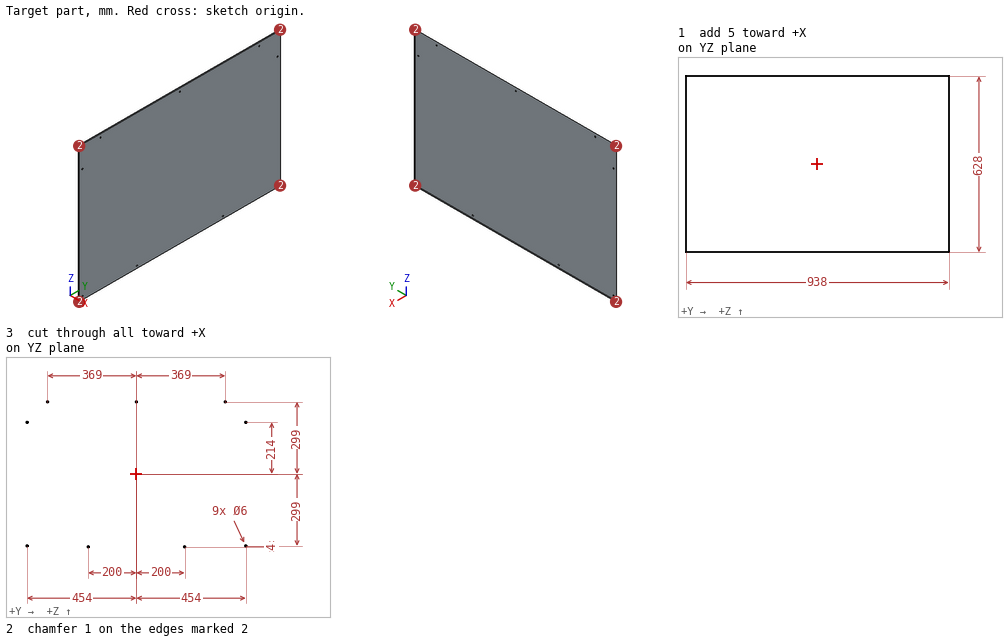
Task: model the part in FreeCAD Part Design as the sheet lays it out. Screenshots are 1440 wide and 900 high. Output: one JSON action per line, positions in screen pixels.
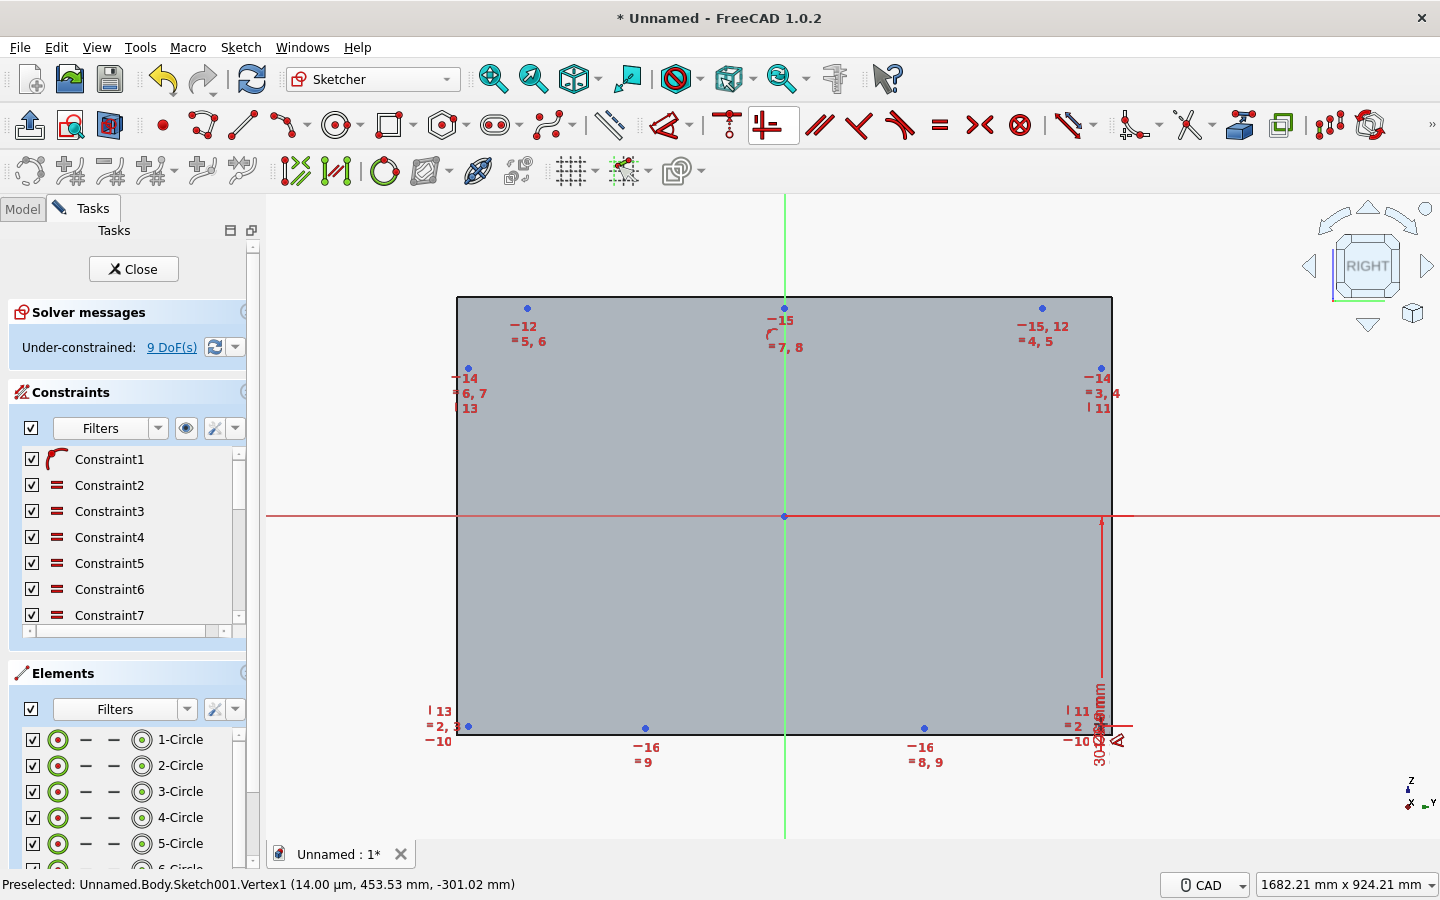
{"action": "scroll", "coordinate": [924, 728], "scroll_direction": "up", "scroll_amount": 14}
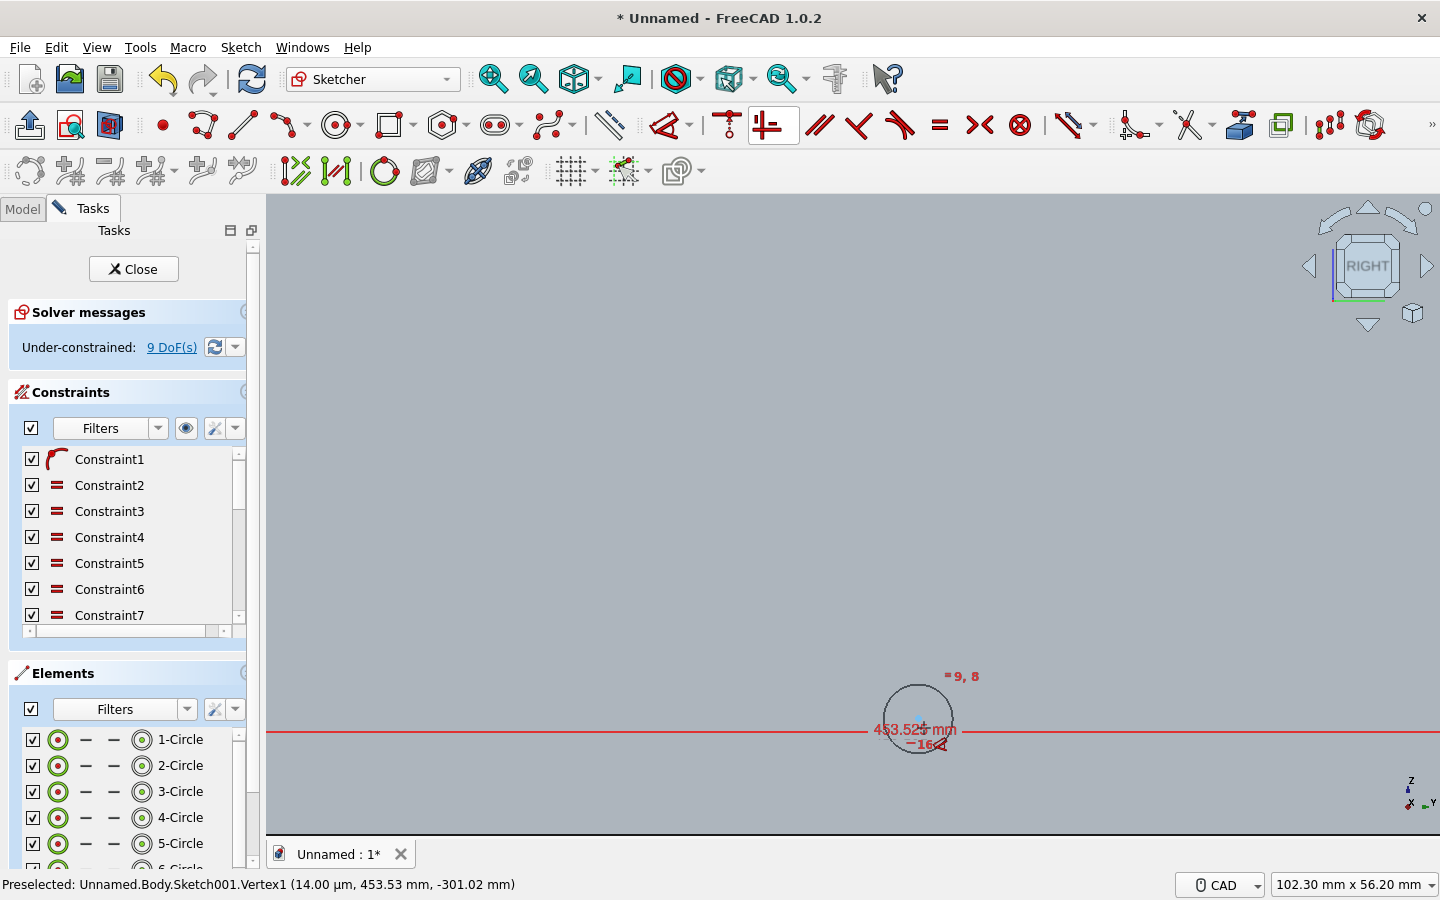
{"action": "left_click", "coordinate": [918, 719]}
{"action": "left_click", "coordinate": [860, 702]}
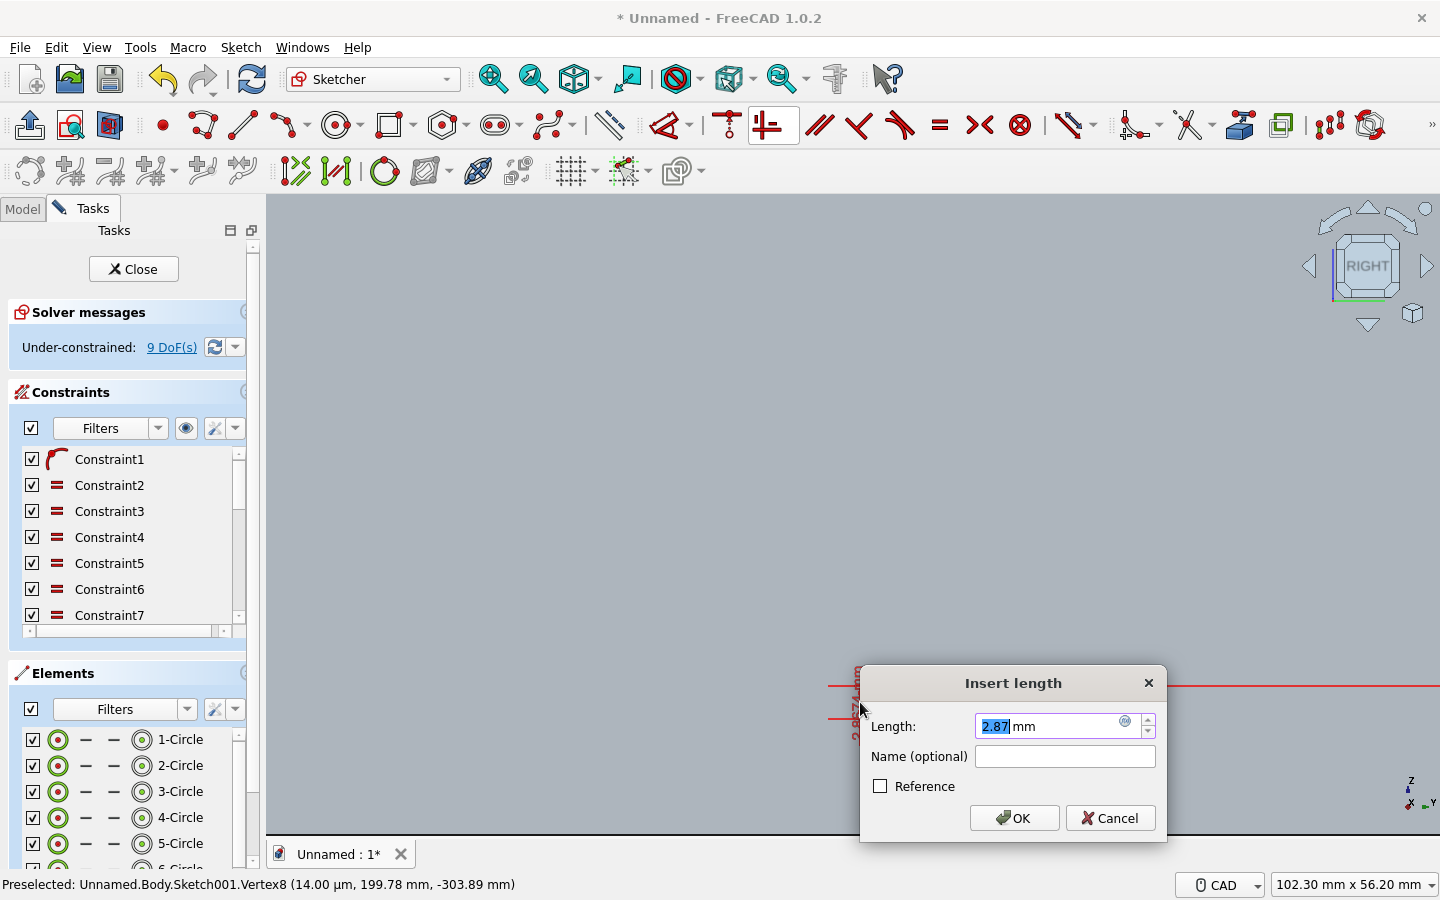
{"action": "type", "text": "4"}
{"action": "key", "text": "Return"}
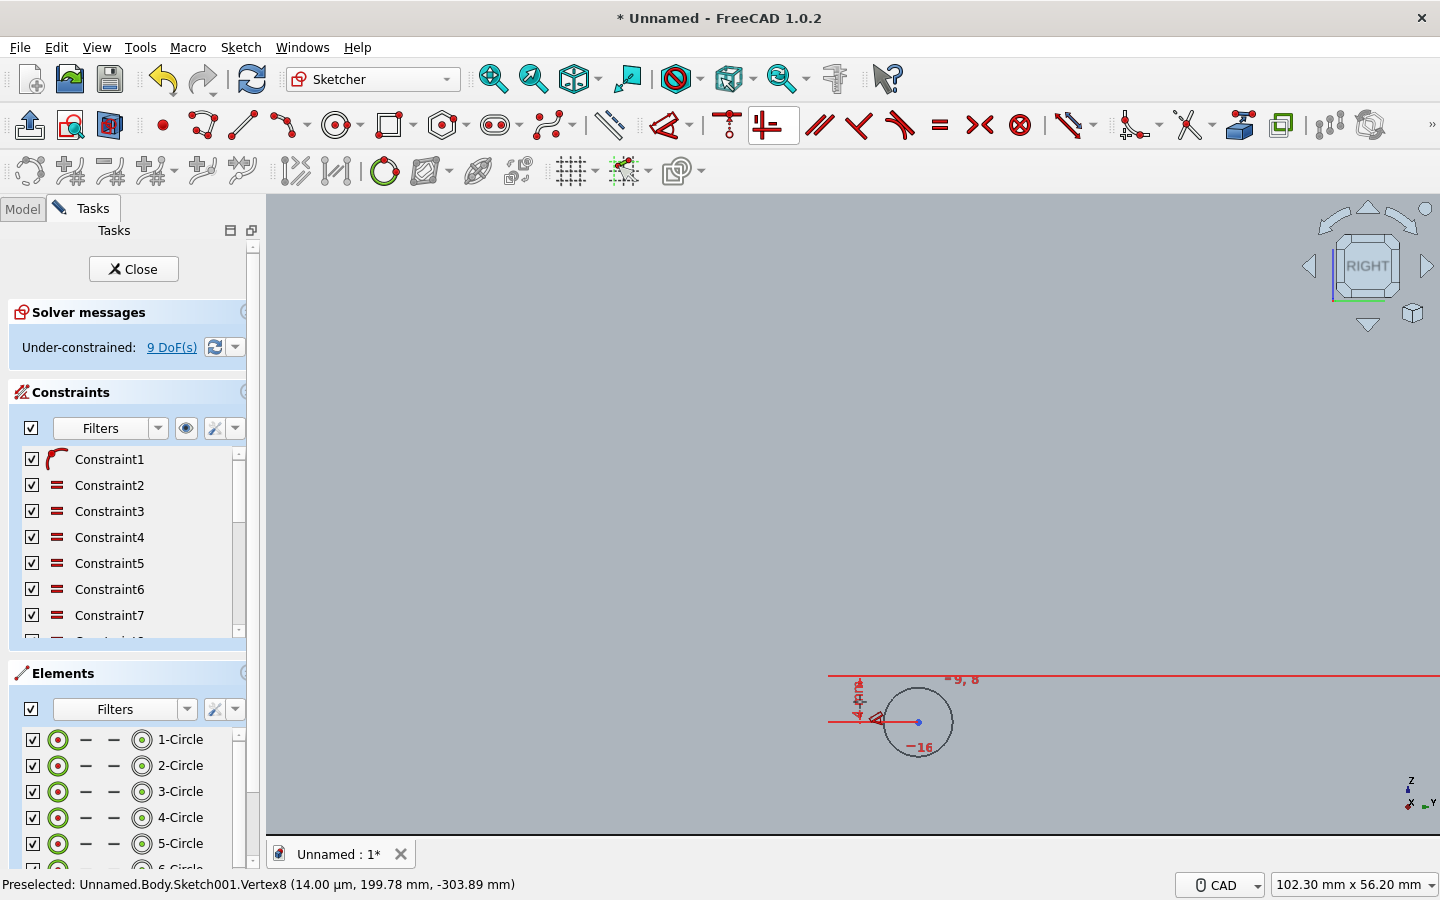
{"action": "scroll", "coordinate": [924, 728], "scroll_direction": "down", "scroll_amount": 14}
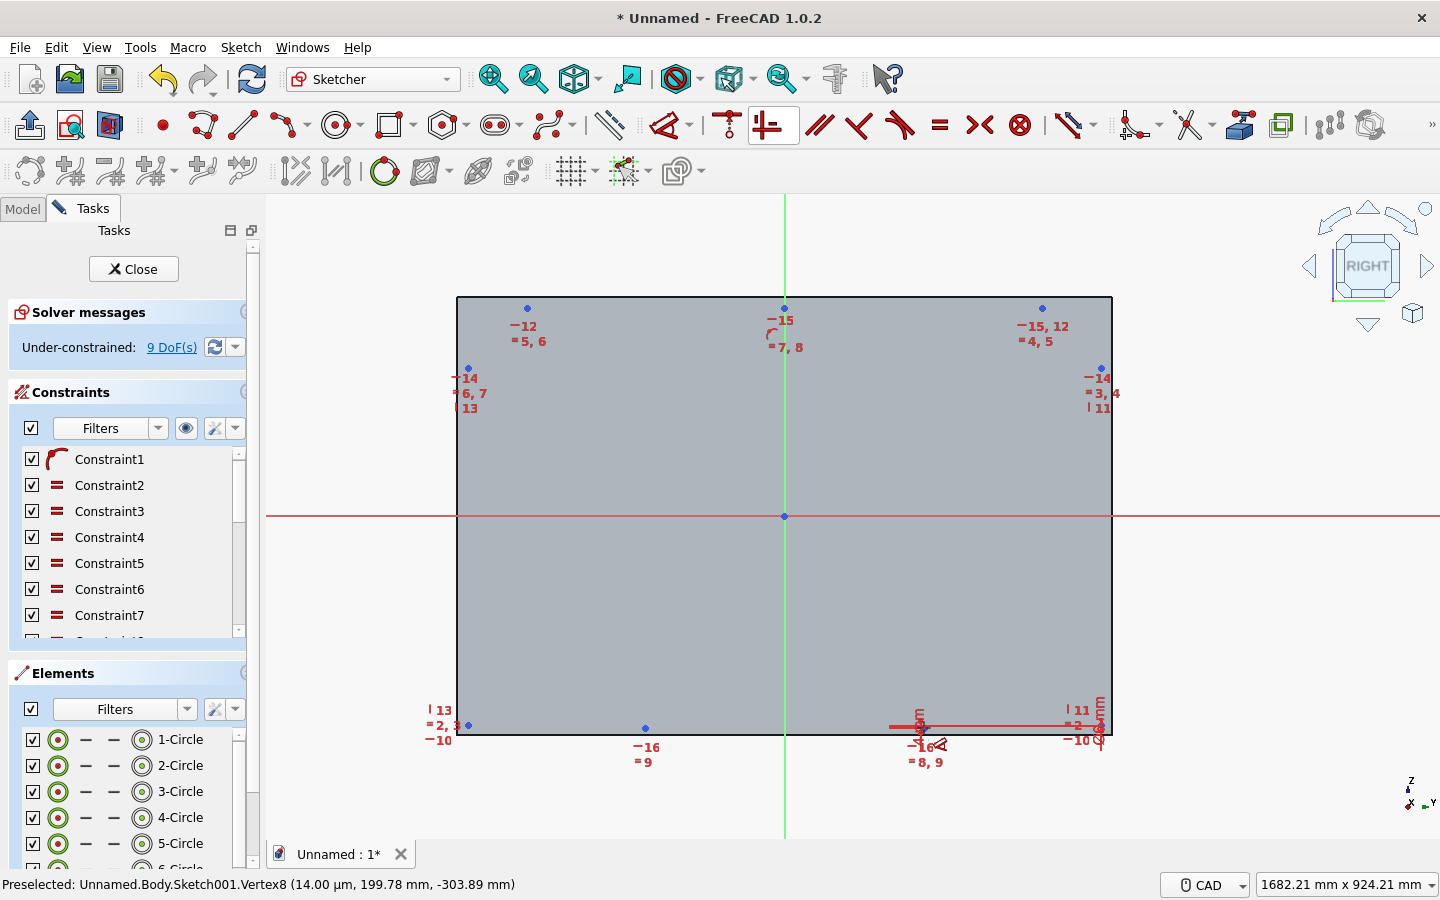
{"action": "left_click", "coordinate": [1101, 726]}
{"action": "left_click", "coordinate": [943, 760]}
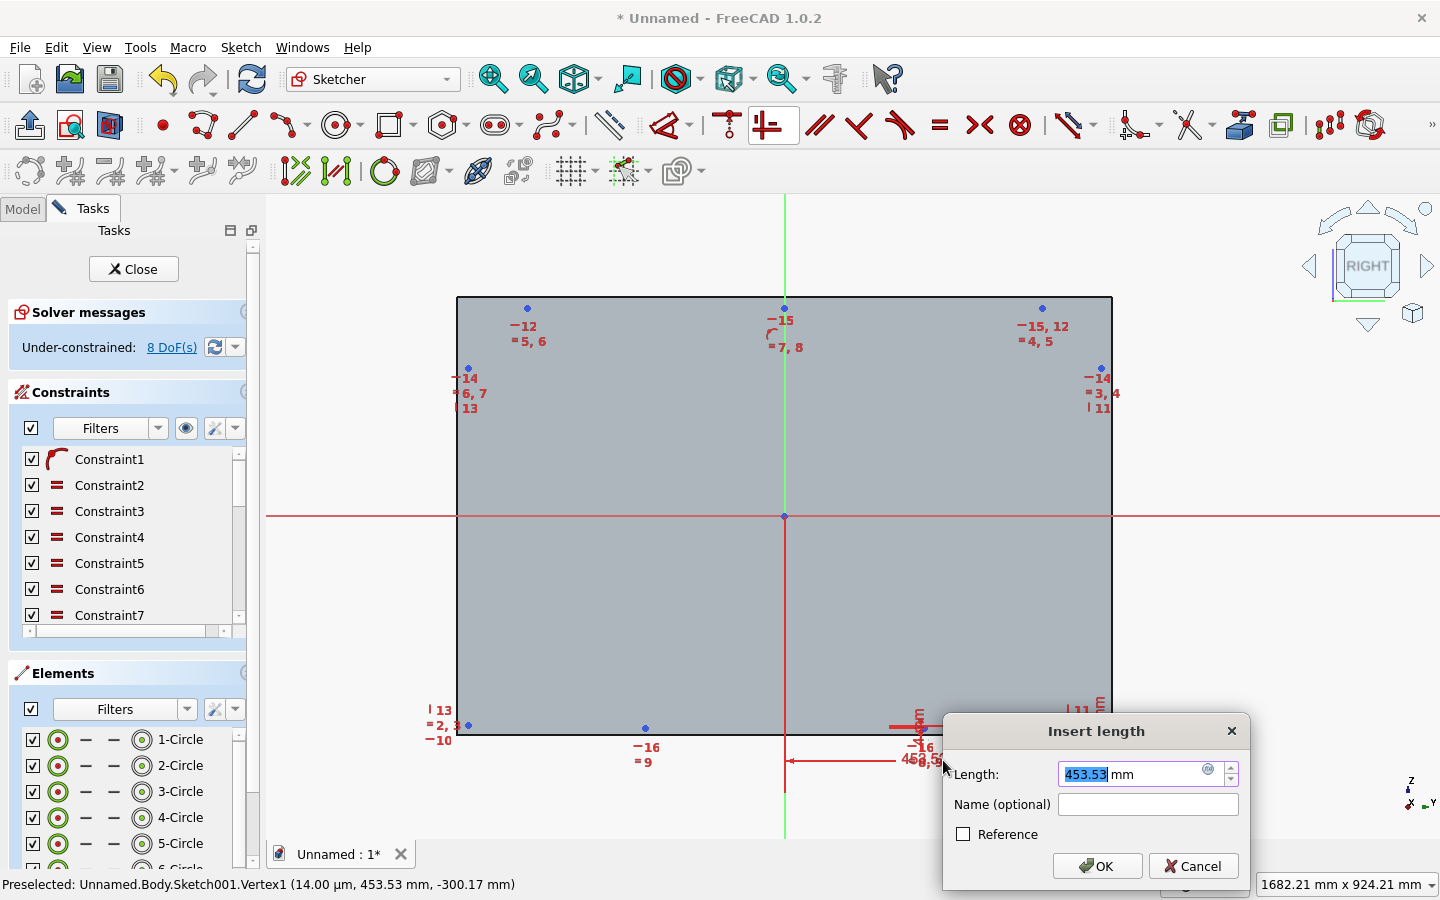
{"action": "type", "text": "454"}
{"action": "key", "text": "Return"}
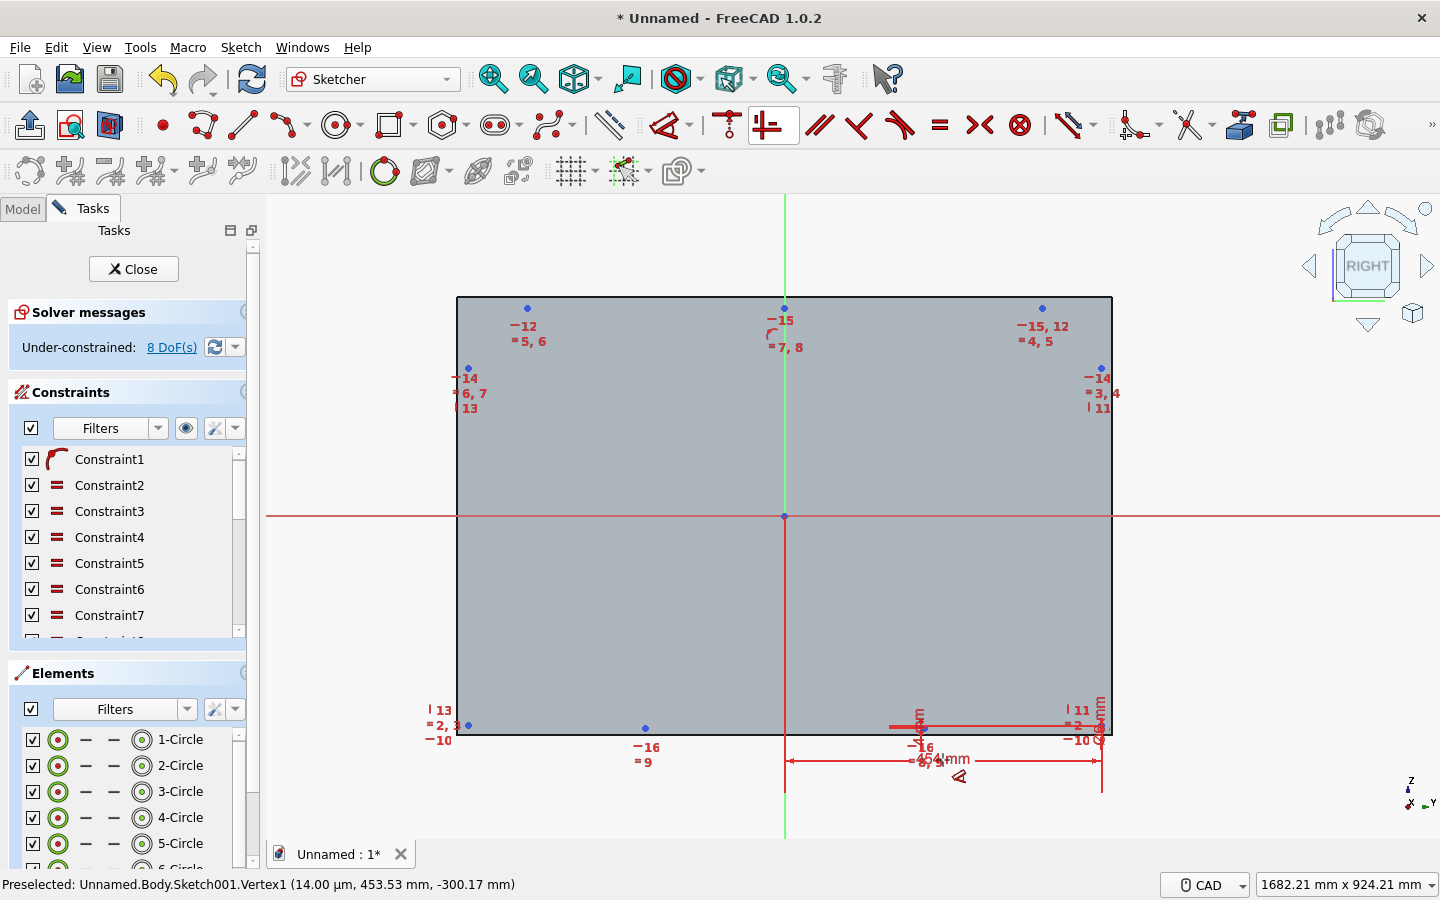
{"action": "left_click", "coordinate": [1102, 726]}
{"action": "left_click", "coordinate": [1136, 621]}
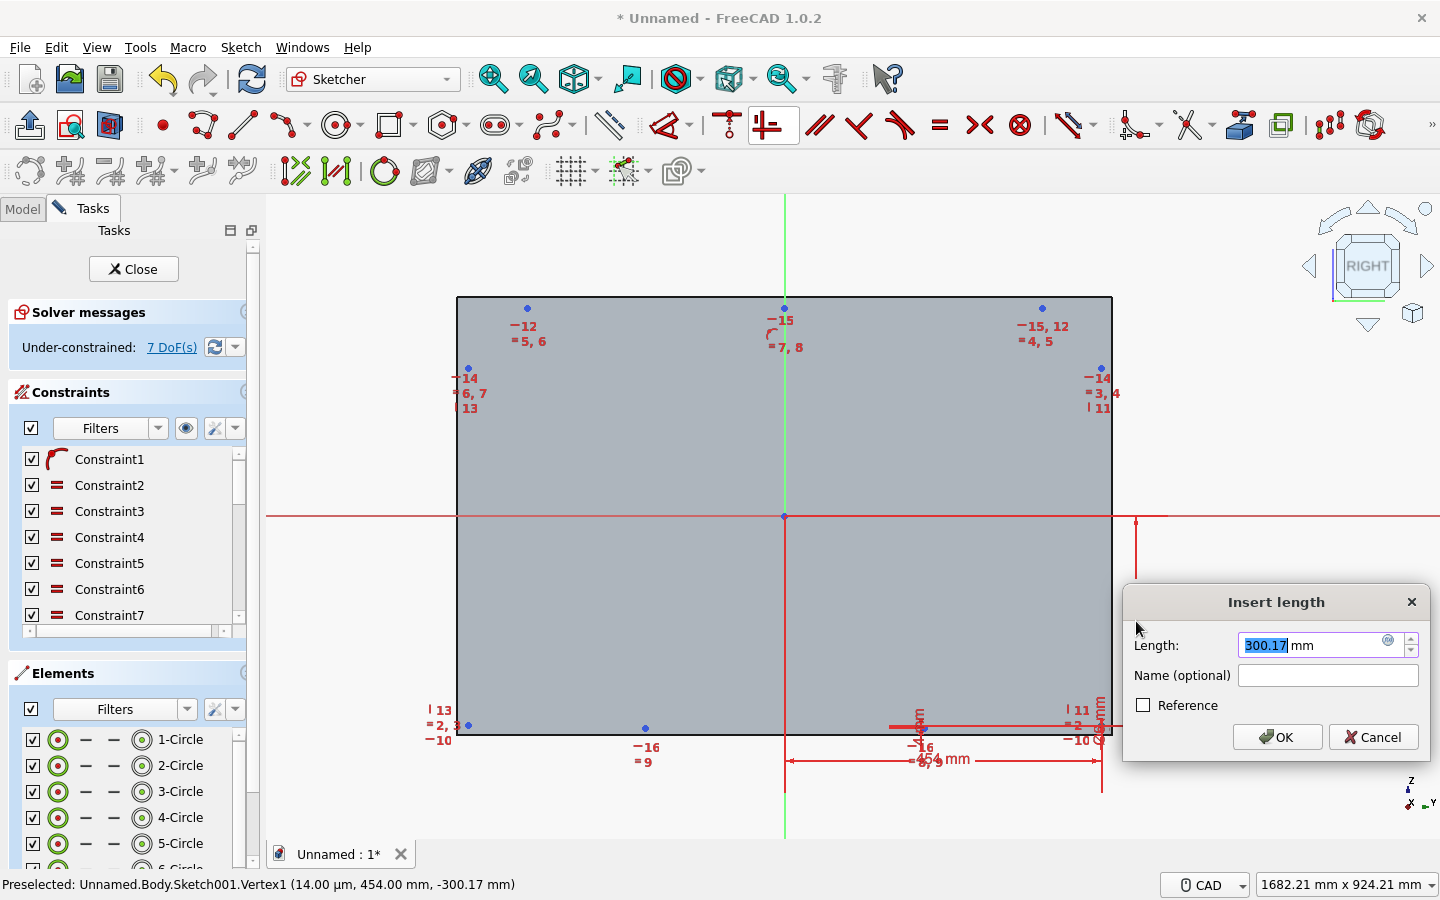
{"action": "type", "text": "299"}
{"action": "key", "text": "Return"}